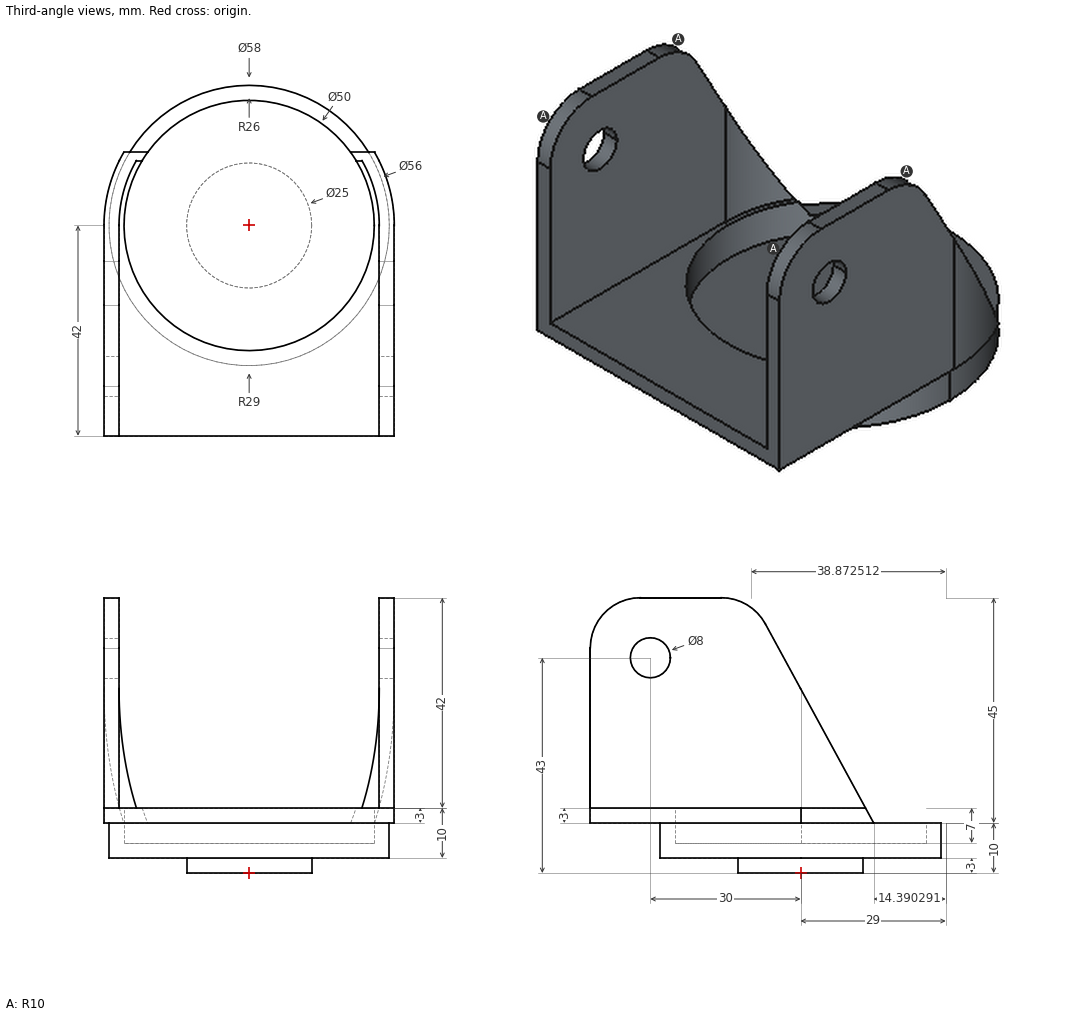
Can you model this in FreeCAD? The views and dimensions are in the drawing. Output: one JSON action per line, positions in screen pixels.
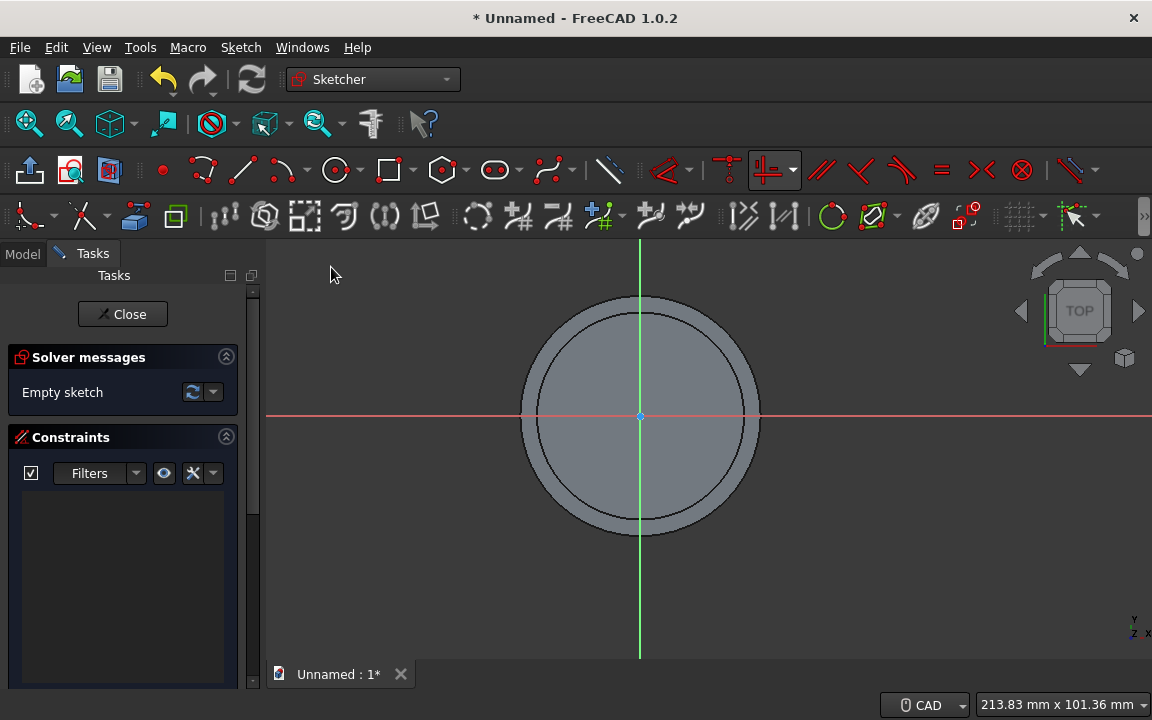
{"action": "scroll", "coordinate": [640, 613], "scroll_direction": "up", "scroll_amount": 2}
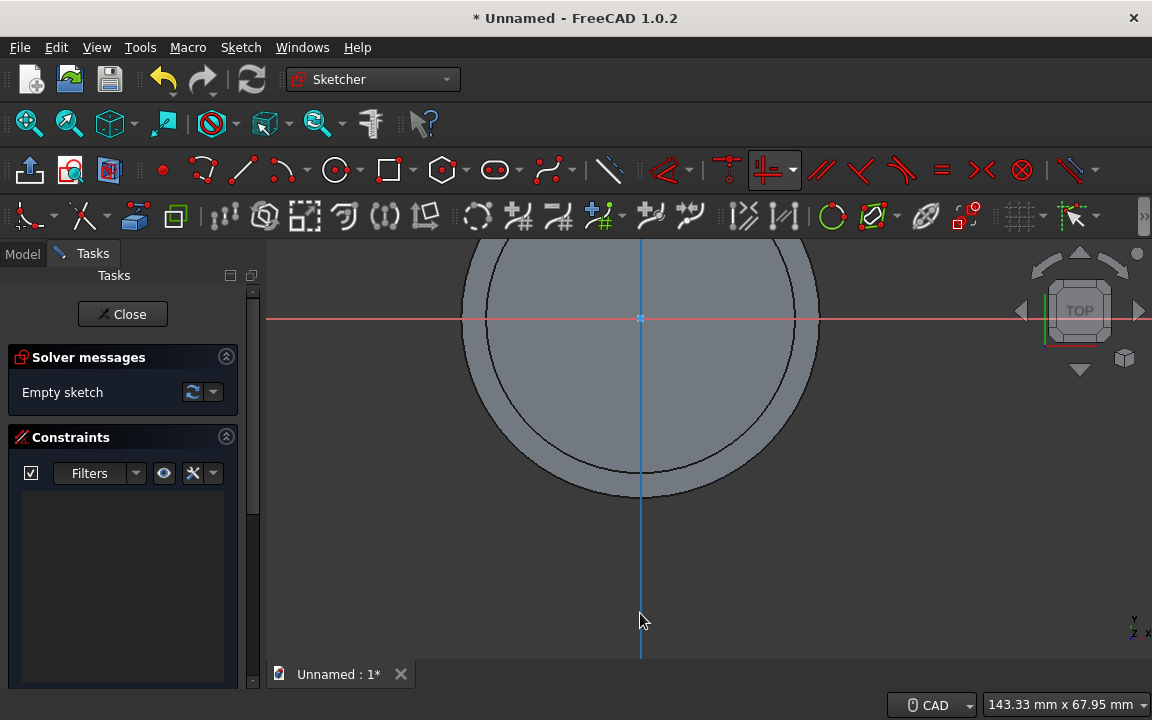
{"action": "left_click", "coordinate": [204, 170]}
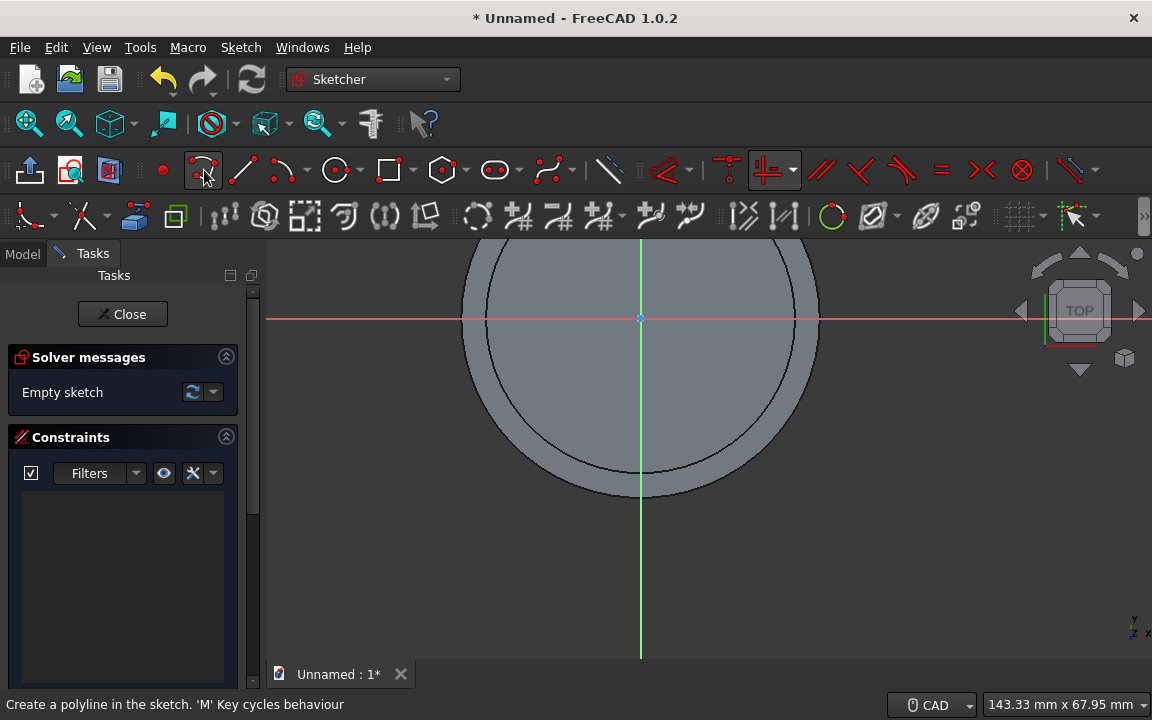
{"action": "left_click", "coordinate": [461, 319]}
{"action": "left_click", "coordinate": [461, 578]}
{"action": "left_click", "coordinate": [820, 578]}
{"action": "left_click", "coordinate": [820, 319]}
{"action": "right_click", "coordinate": [820, 319]}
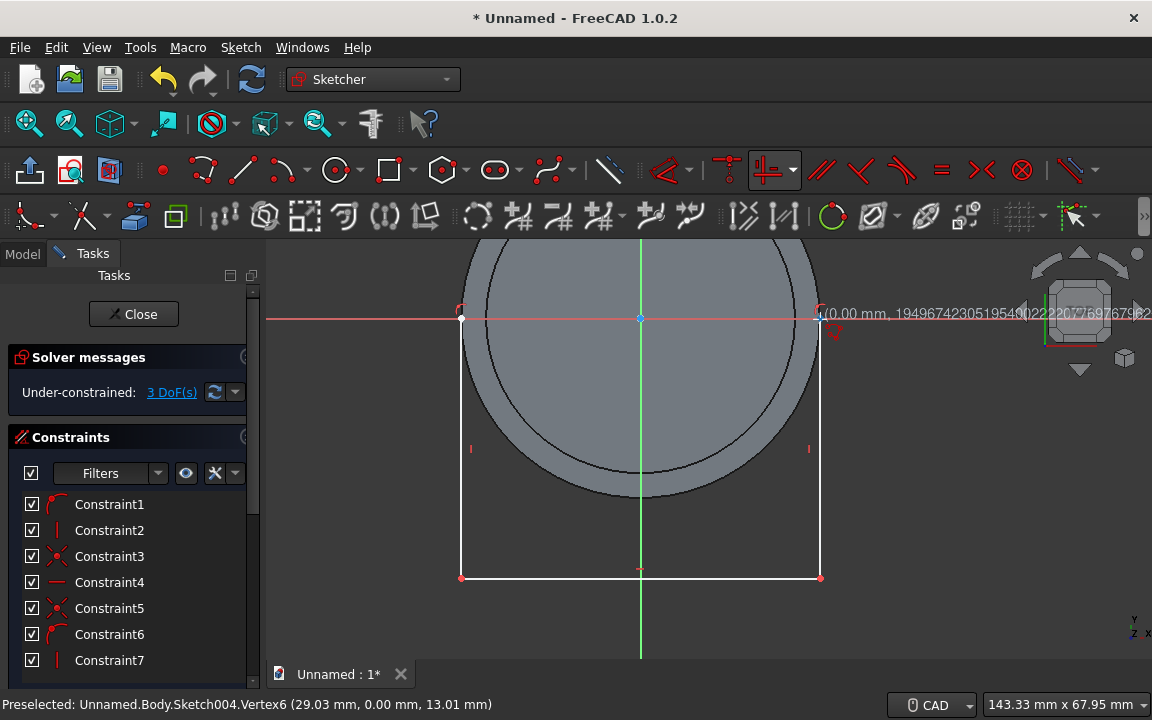
{"action": "left_click", "coordinate": [310, 170]}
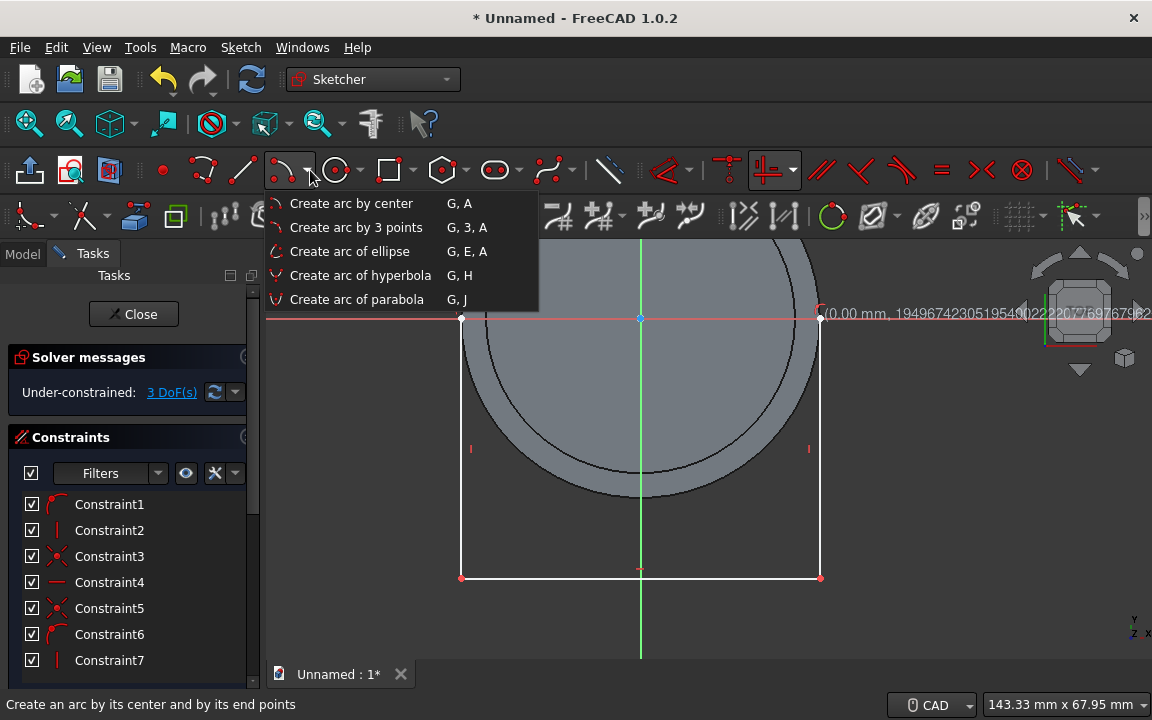
{"action": "left_click", "coordinate": [402, 227]}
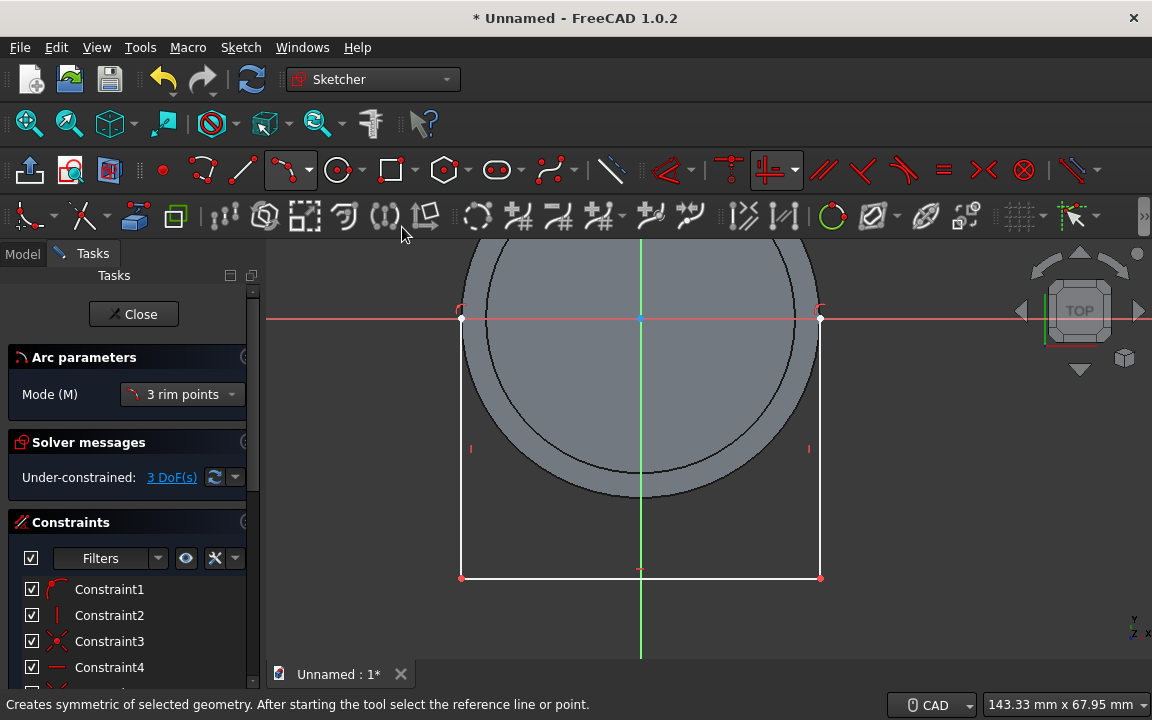
{"action": "left_click", "coordinate": [820, 319]}
{"action": "left_click", "coordinate": [461, 319]}
{"action": "left_click", "coordinate": [585, 489]}
{"action": "key", "text": "Escape"}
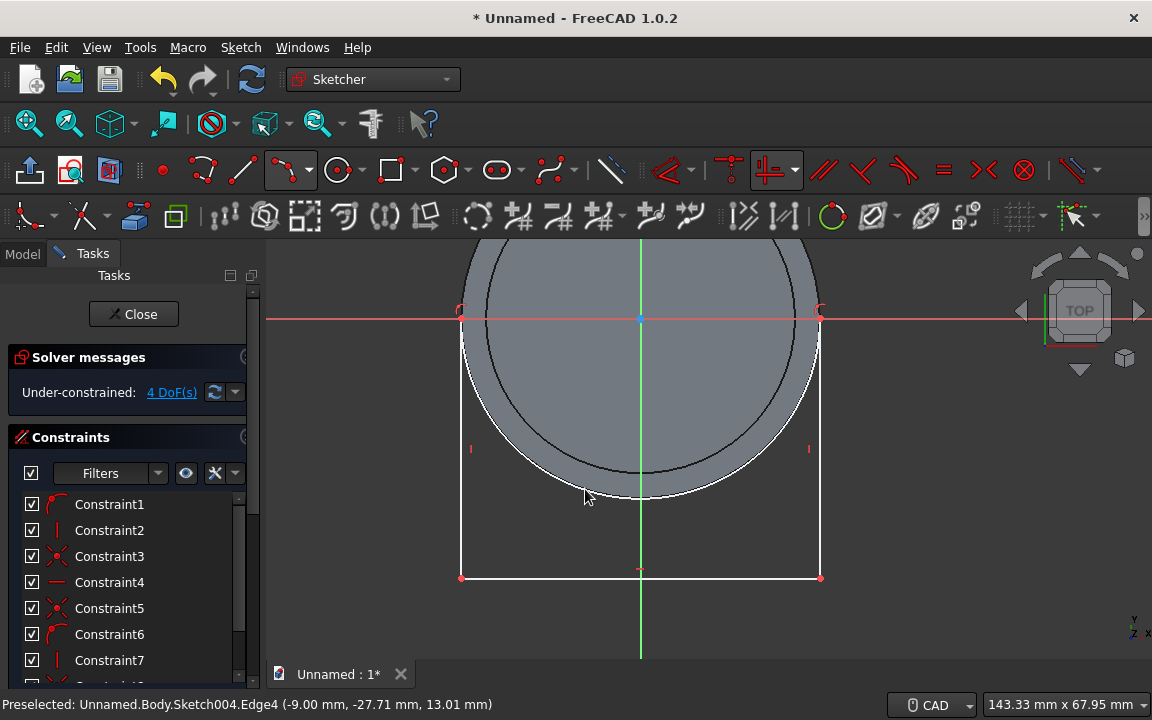
{"action": "left_click_drag", "start_coordinate": [630, 309], "coordinate": [651, 329]}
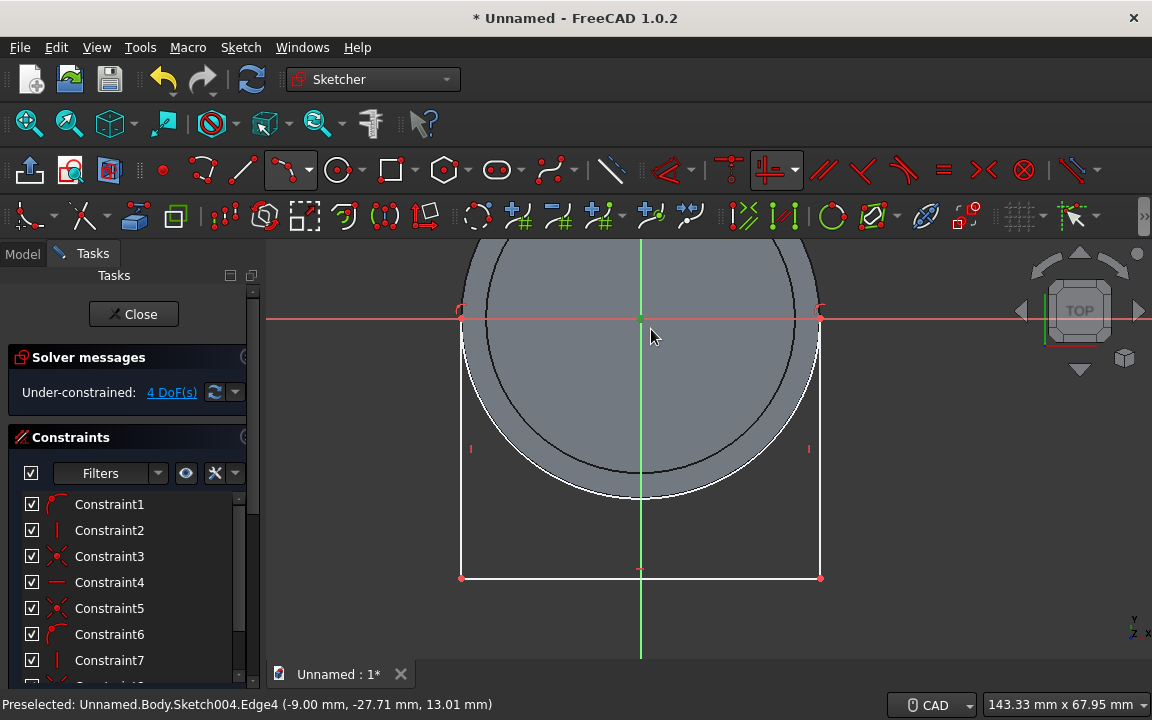
{"action": "left_click", "coordinate": [730, 170]}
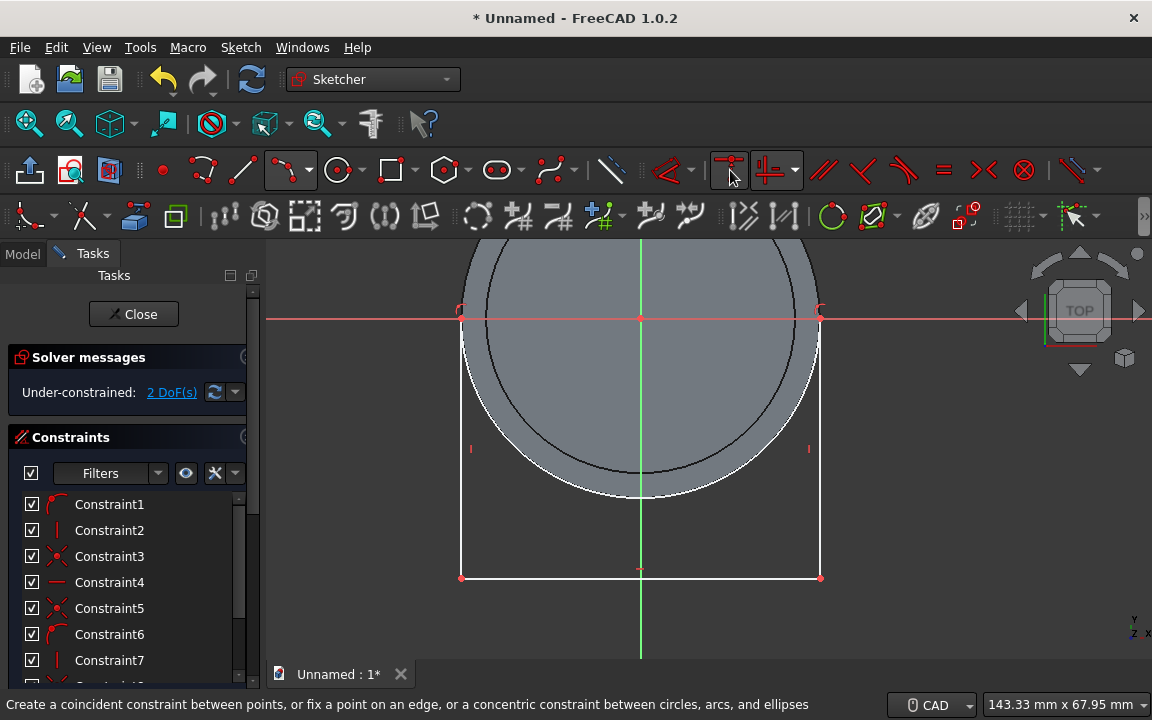
{"action": "left_click", "coordinate": [666, 170]}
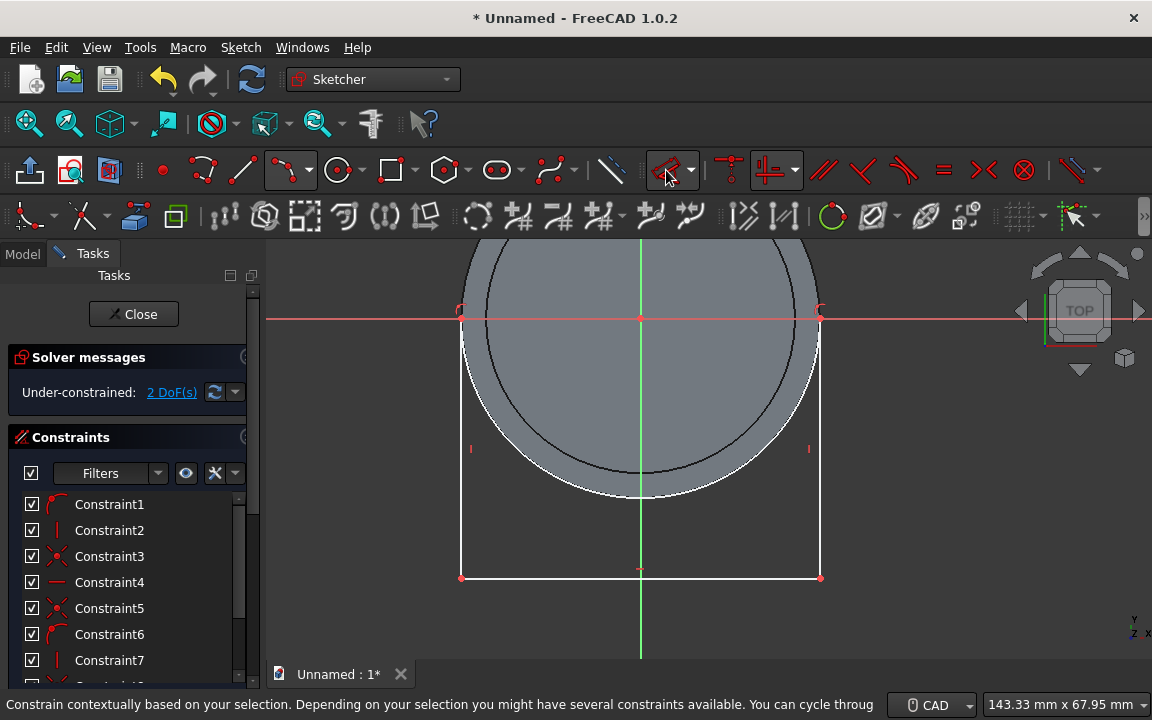
{"action": "left_click", "coordinate": [535, 464]}
{"action": "left_click", "coordinate": [516, 490]}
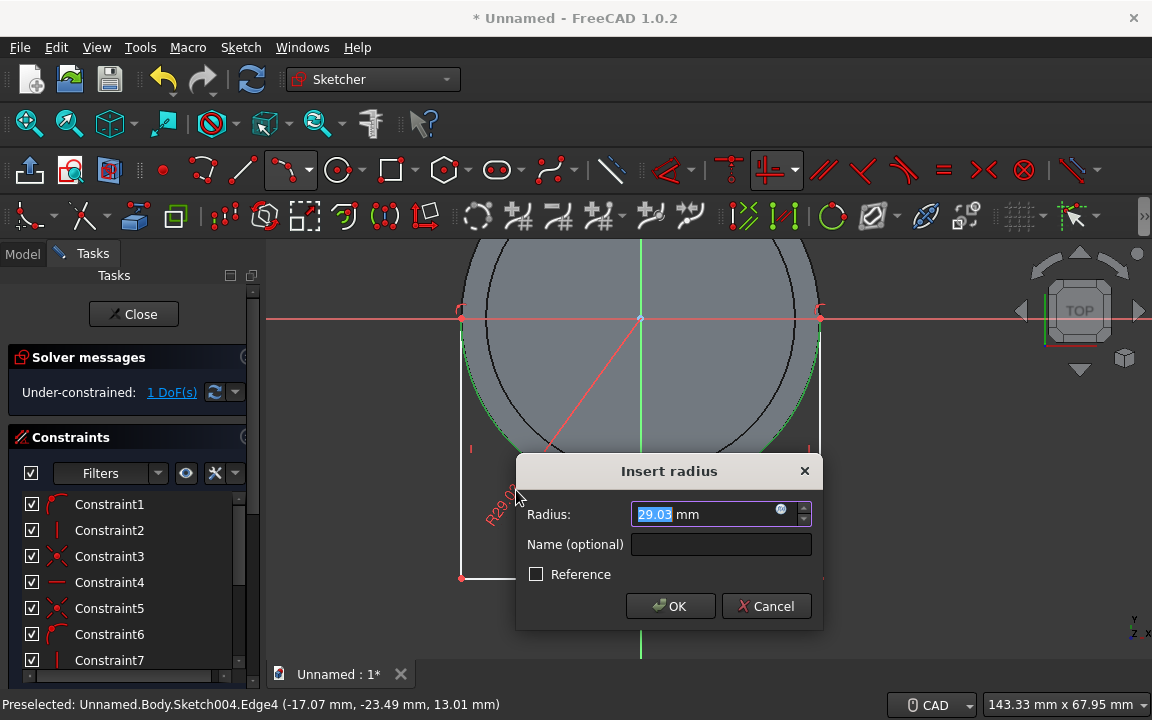
{"action": "type", "text": "29"}
{"action": "key", "text": "Return"}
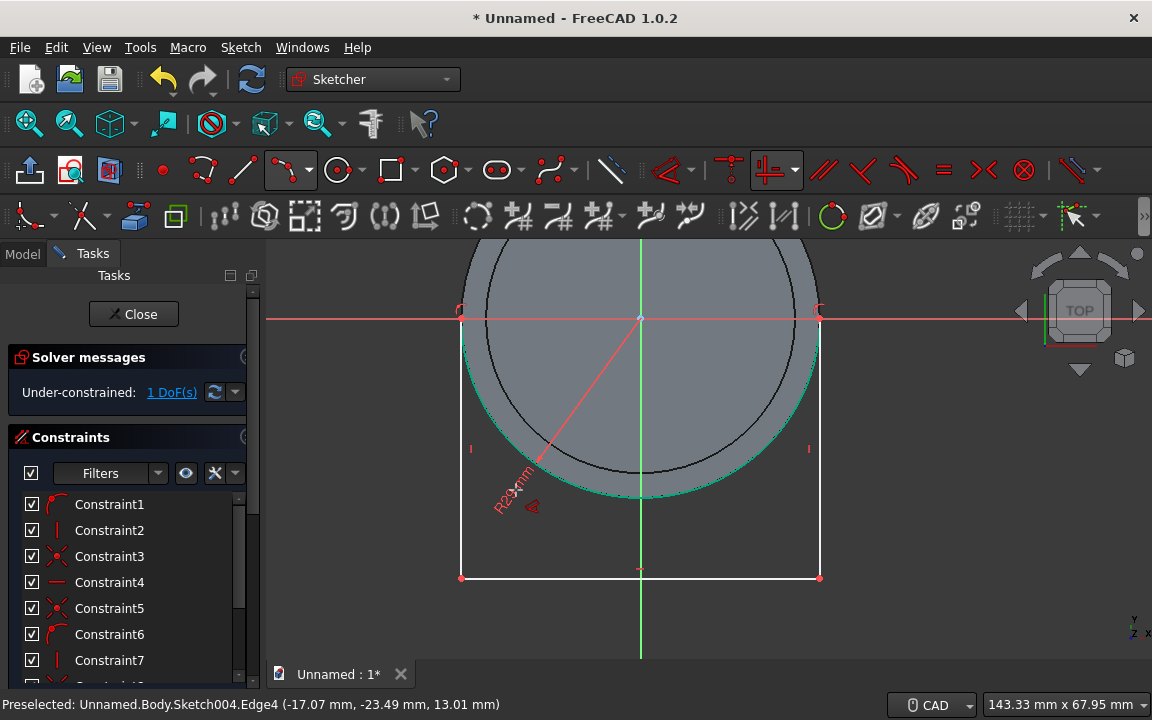
{"action": "left_click", "coordinate": [461, 397]}
{"action": "left_click", "coordinate": [427, 449]}